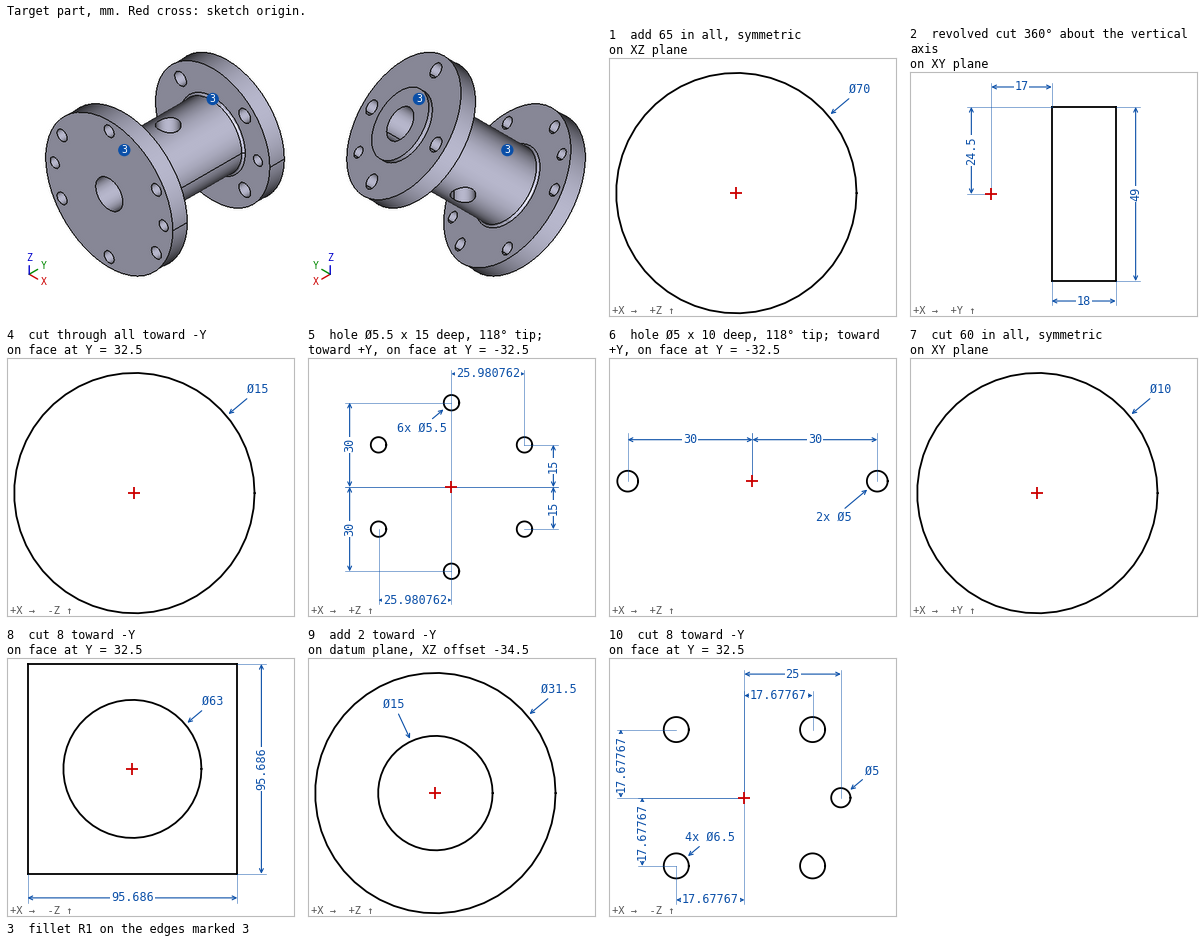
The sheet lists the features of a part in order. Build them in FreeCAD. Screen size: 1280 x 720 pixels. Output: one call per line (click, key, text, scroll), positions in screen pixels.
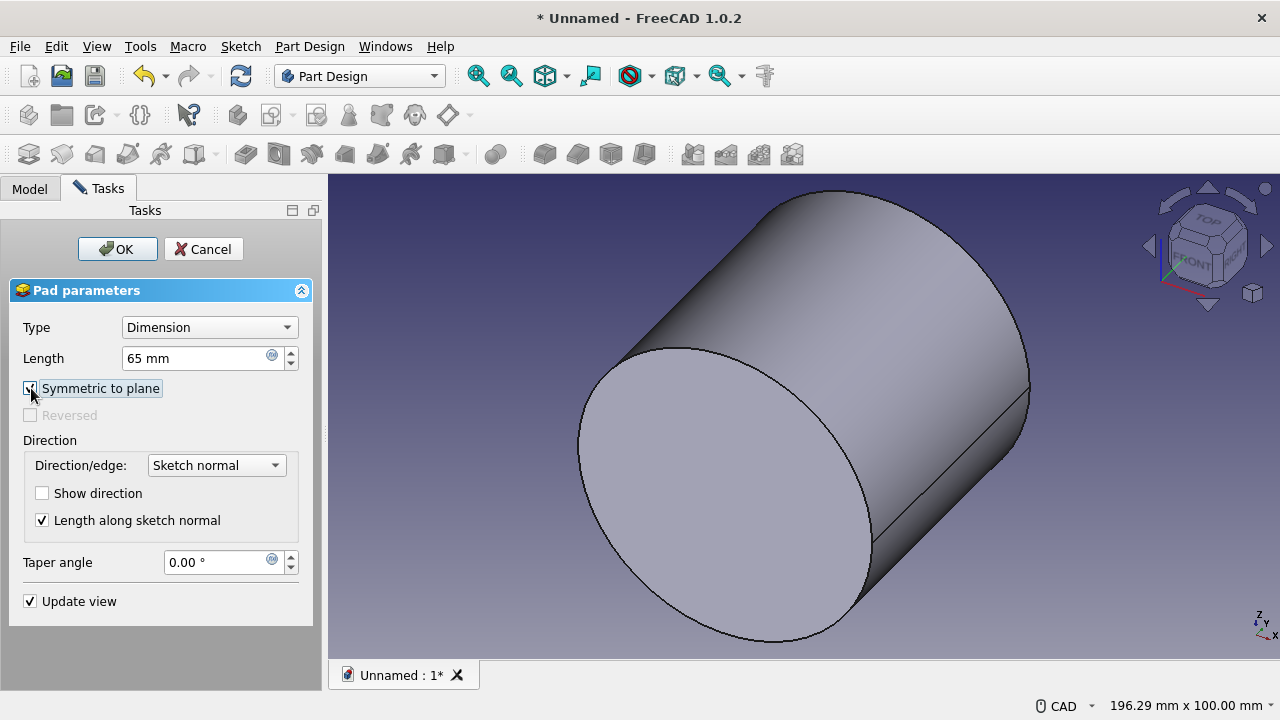
click(118, 249)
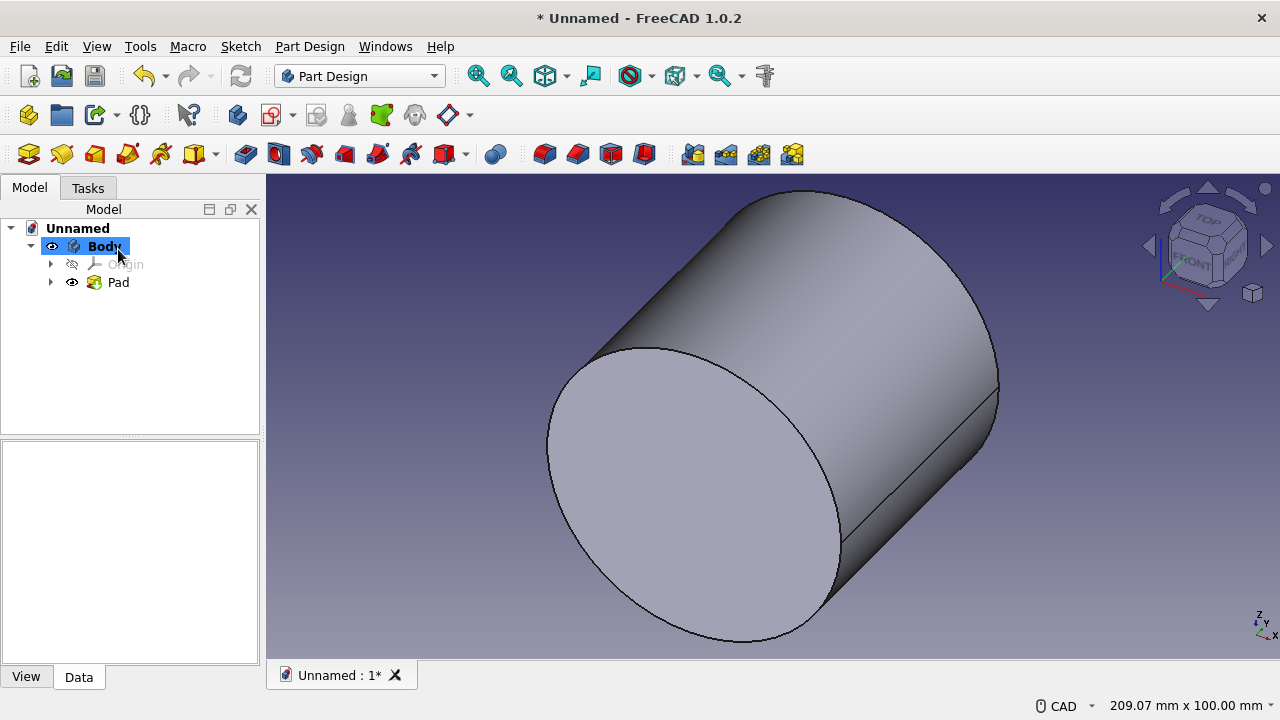
click(479, 76)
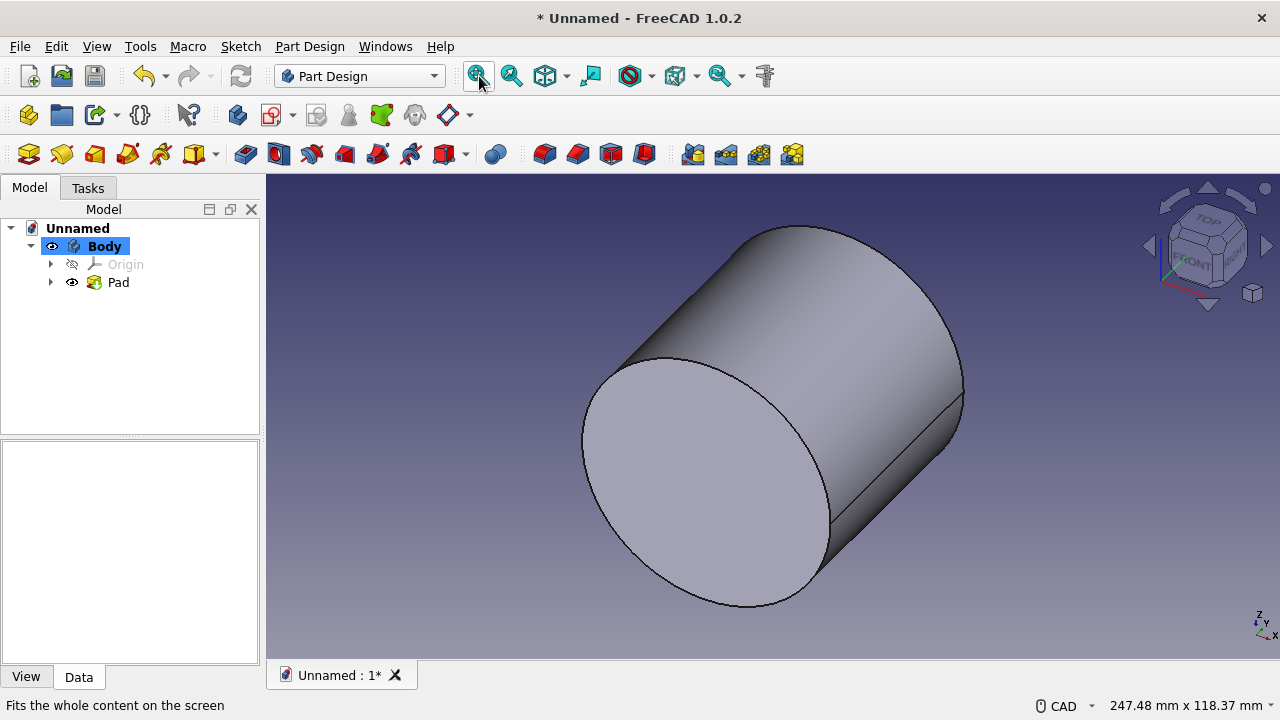
click(270, 116)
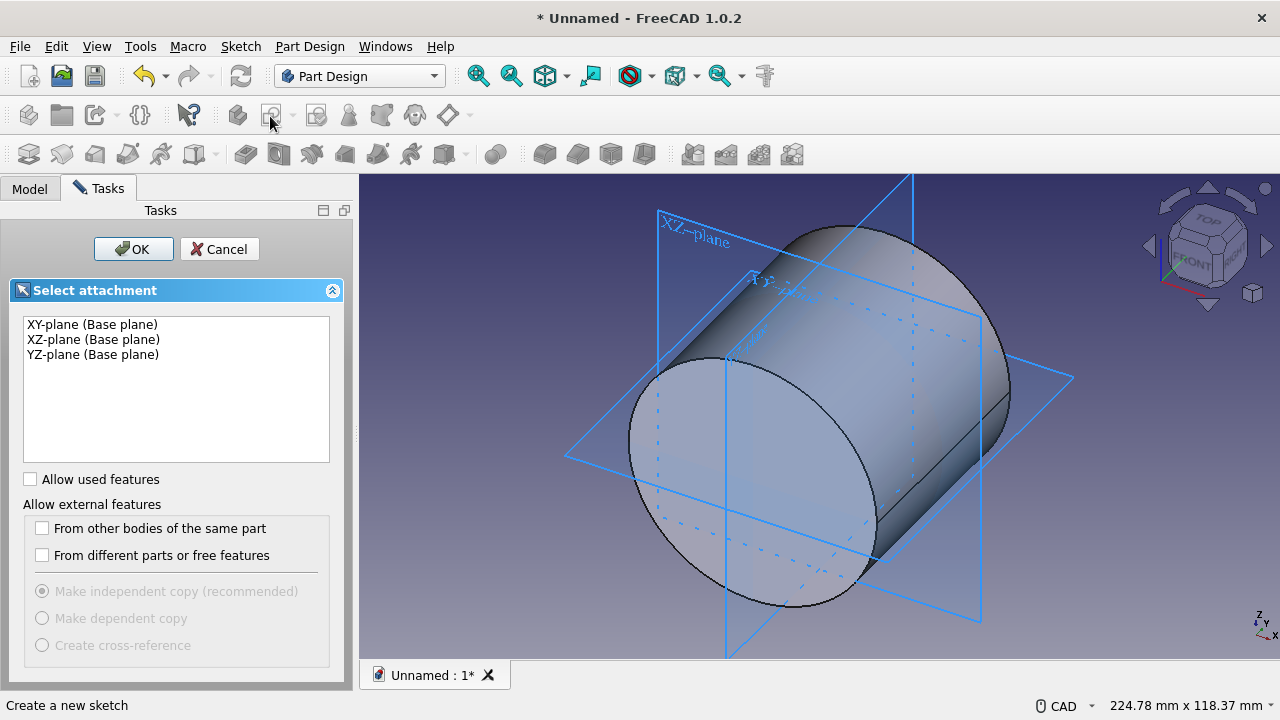
click(84, 324)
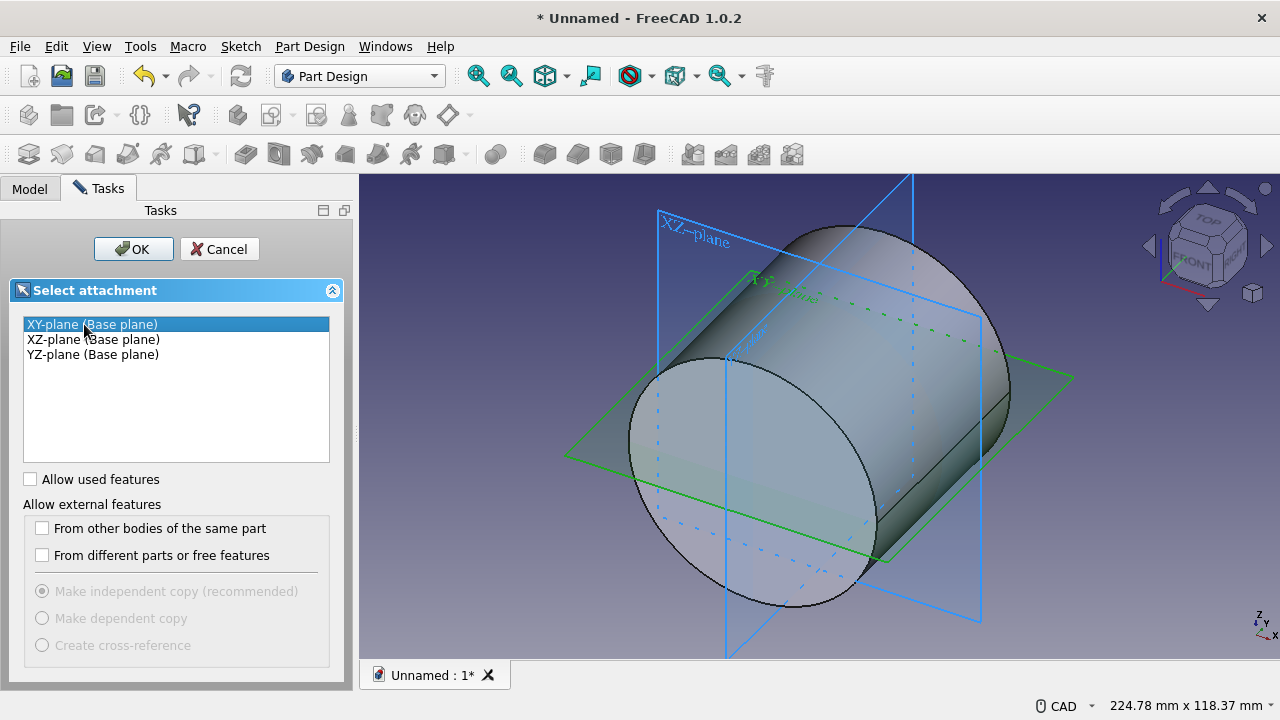
click(134, 249)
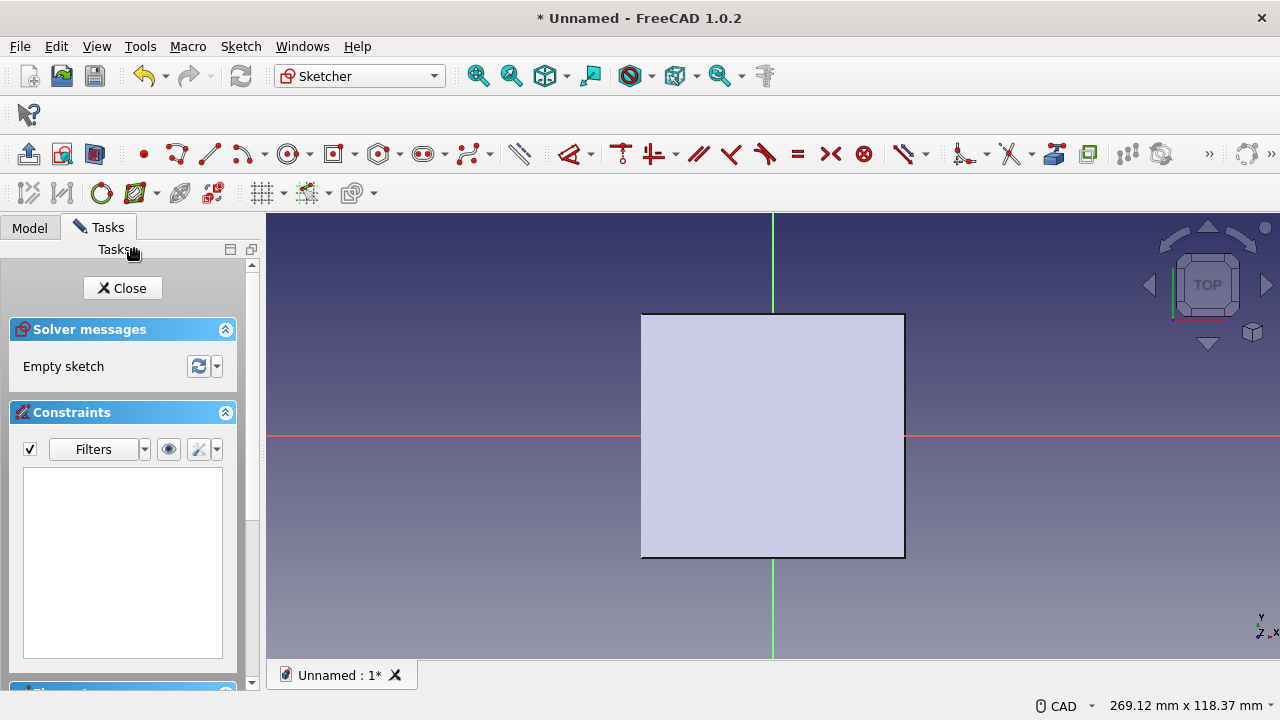
click(95, 154)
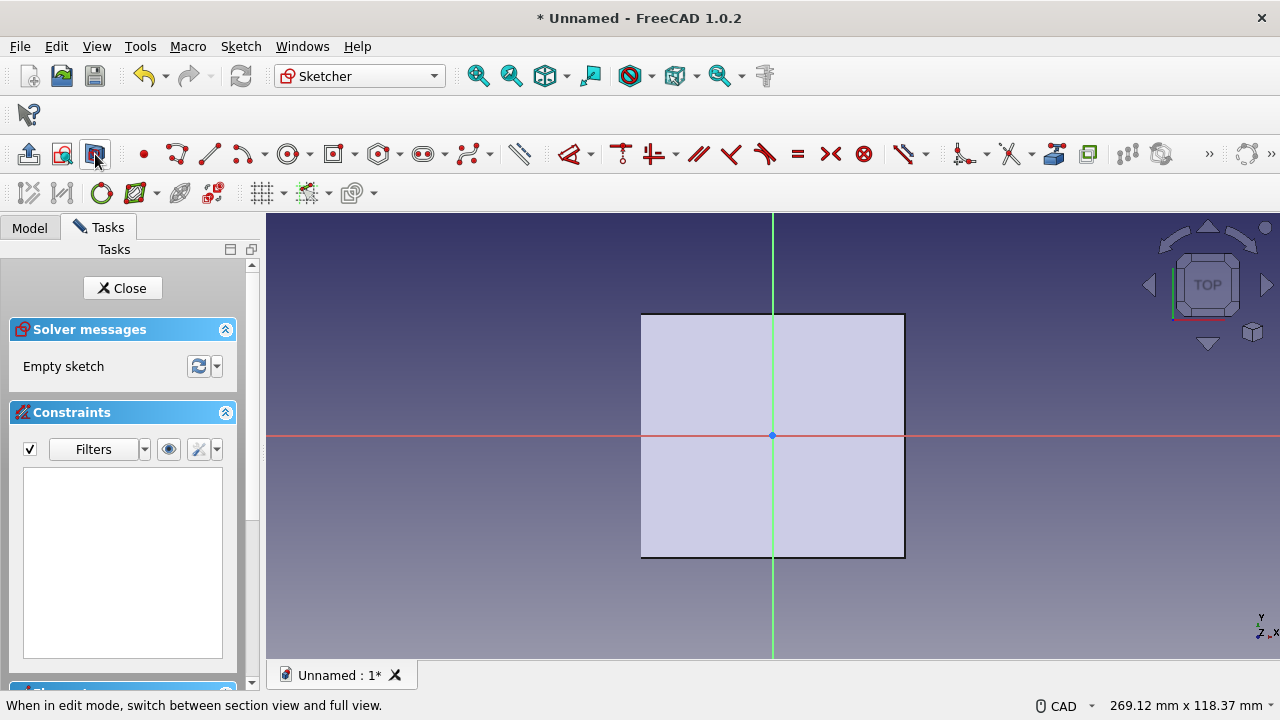
scroll(1112, 436, up, 2)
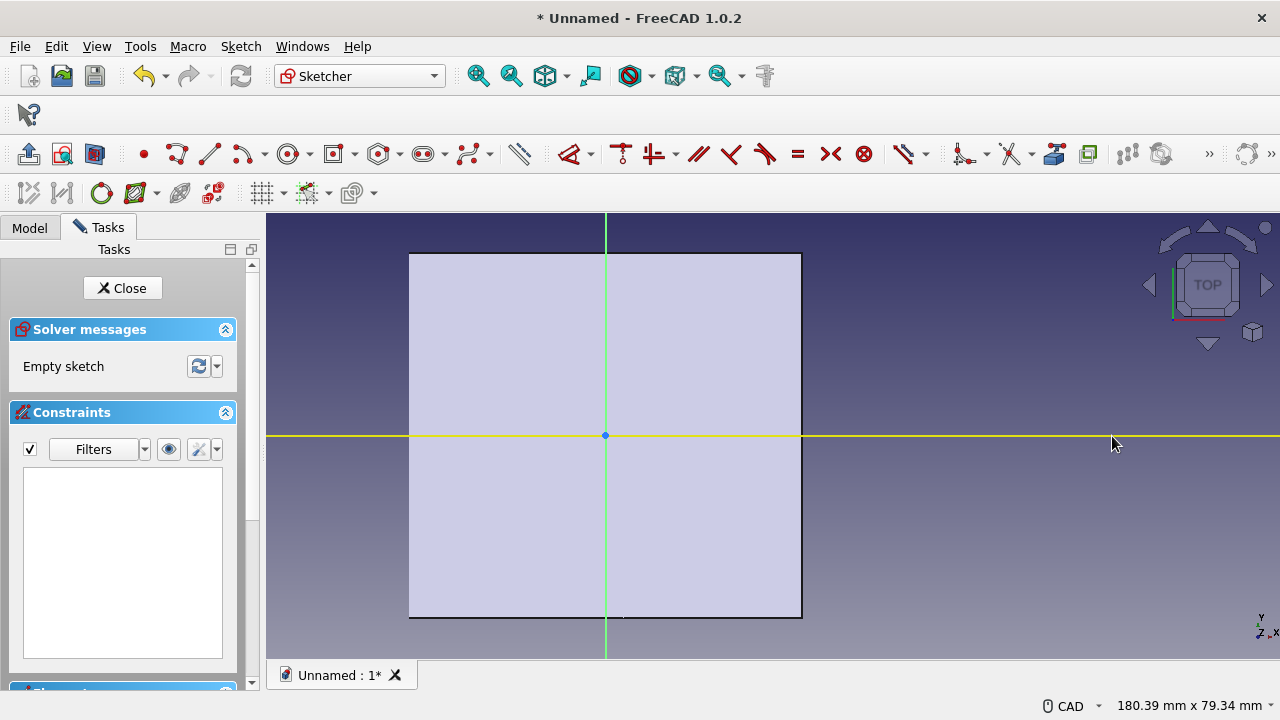
click(354, 154)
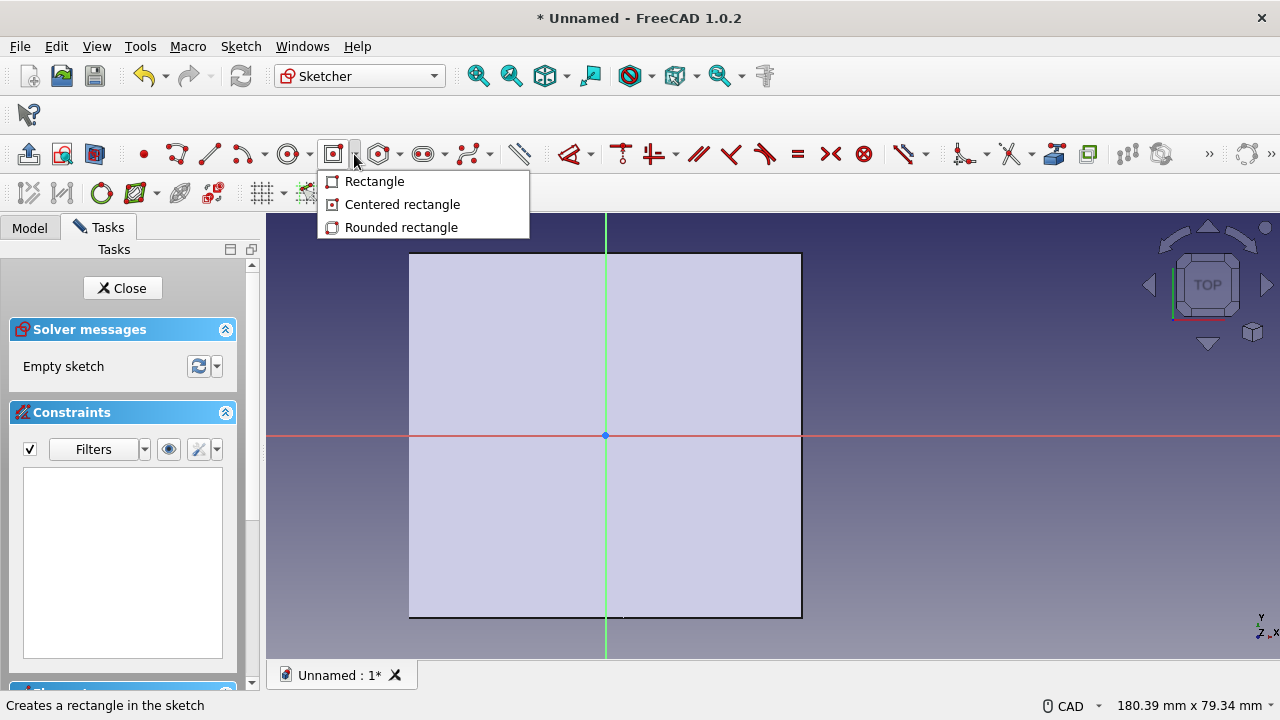
click(424, 182)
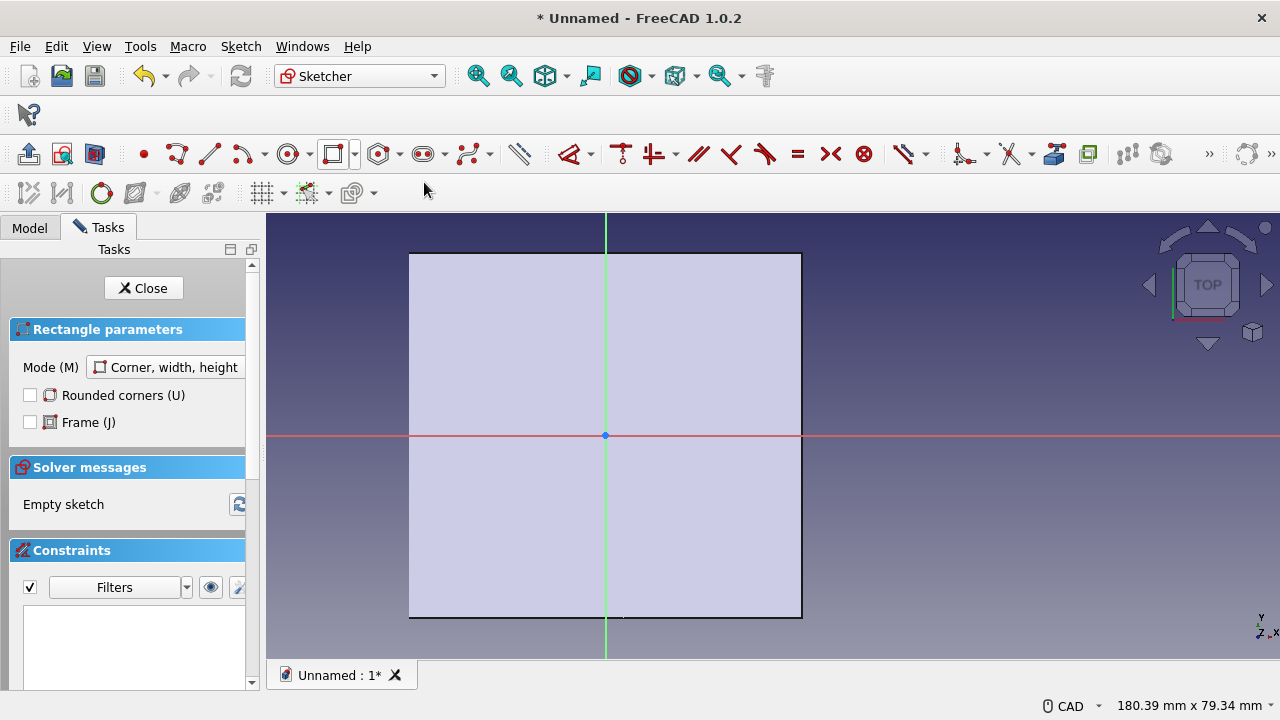
click(701, 298)
move(802, 573)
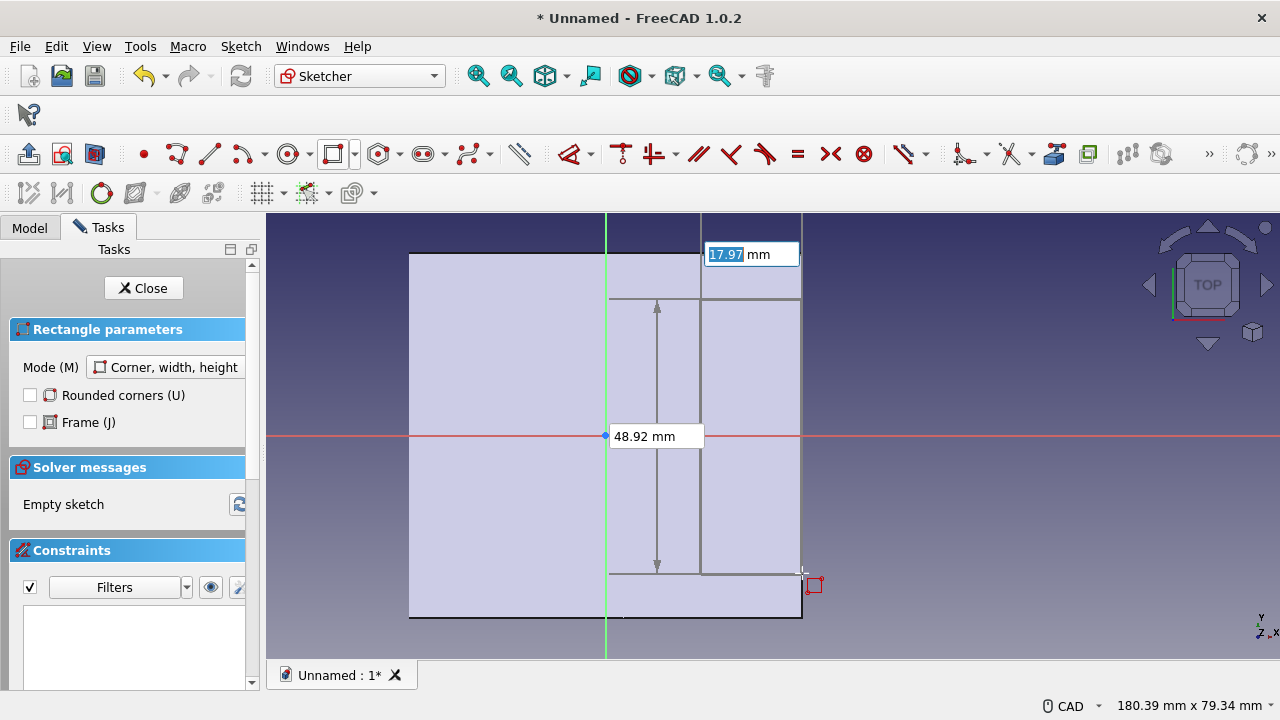
text(18)
key(Tab)
text(49)
key(Return)
key(Escape)